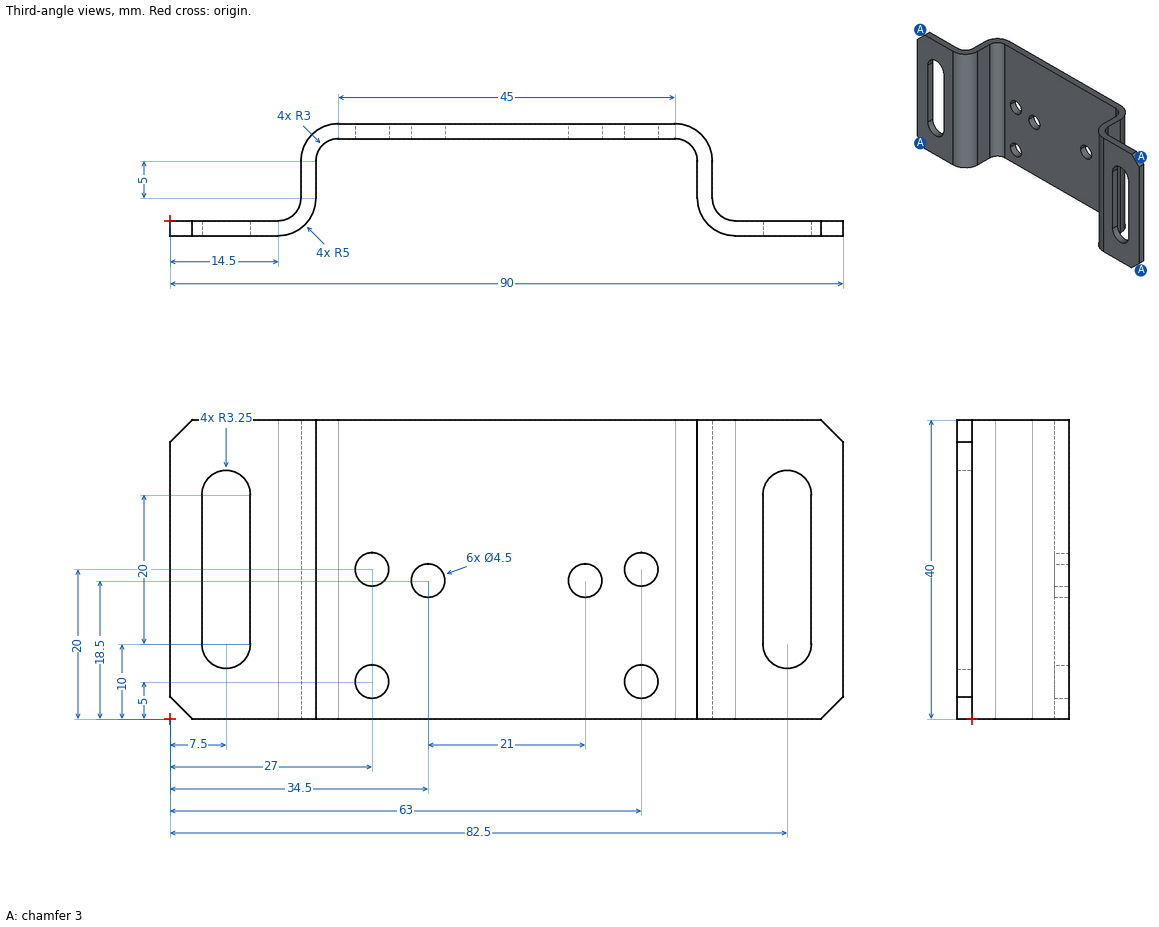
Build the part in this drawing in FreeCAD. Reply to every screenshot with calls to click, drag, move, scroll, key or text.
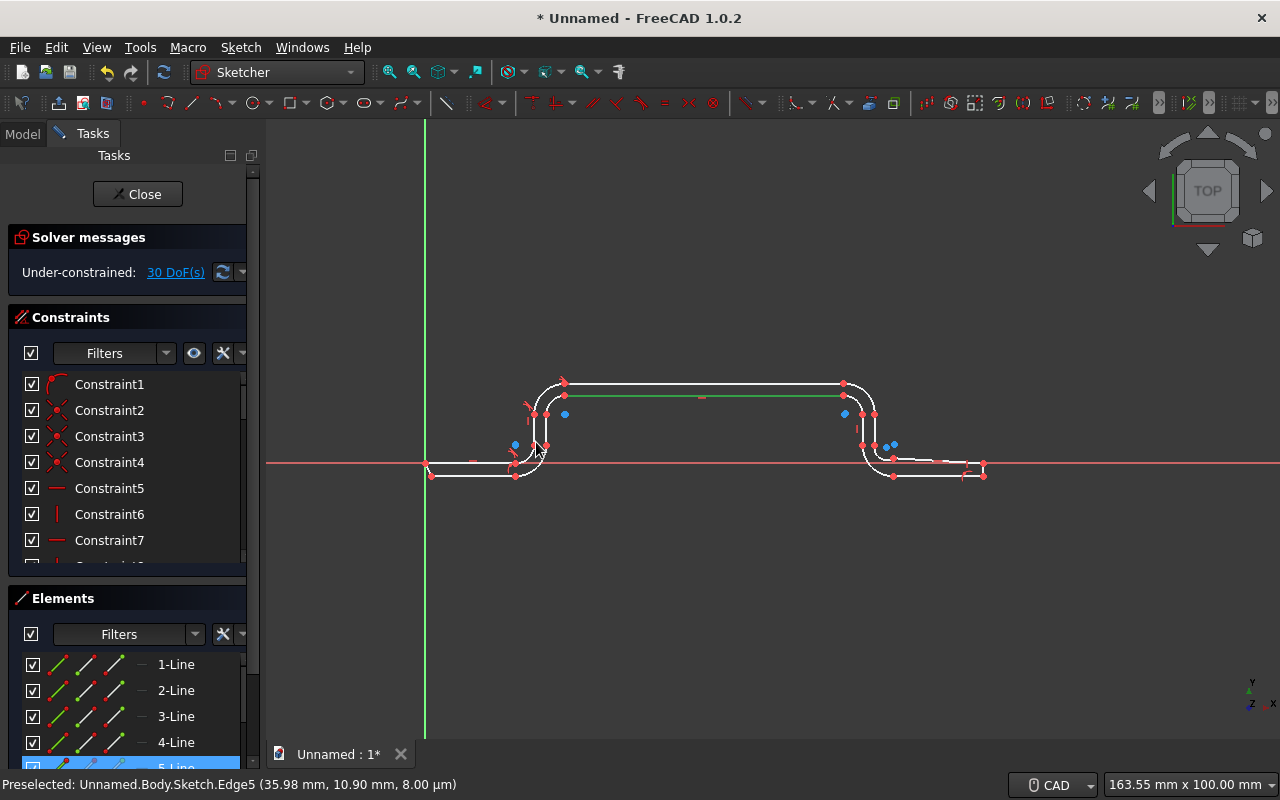
scroll(861, 406, up, 3)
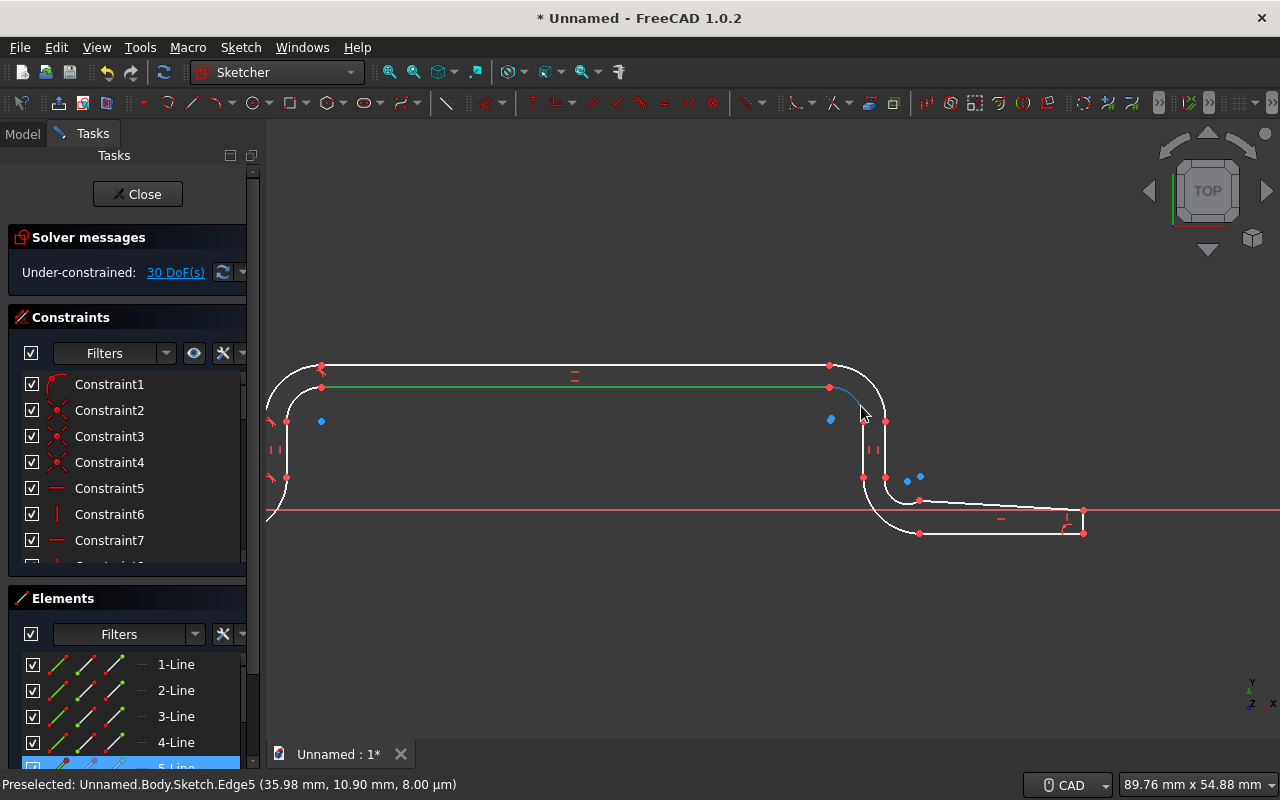
click(860, 406)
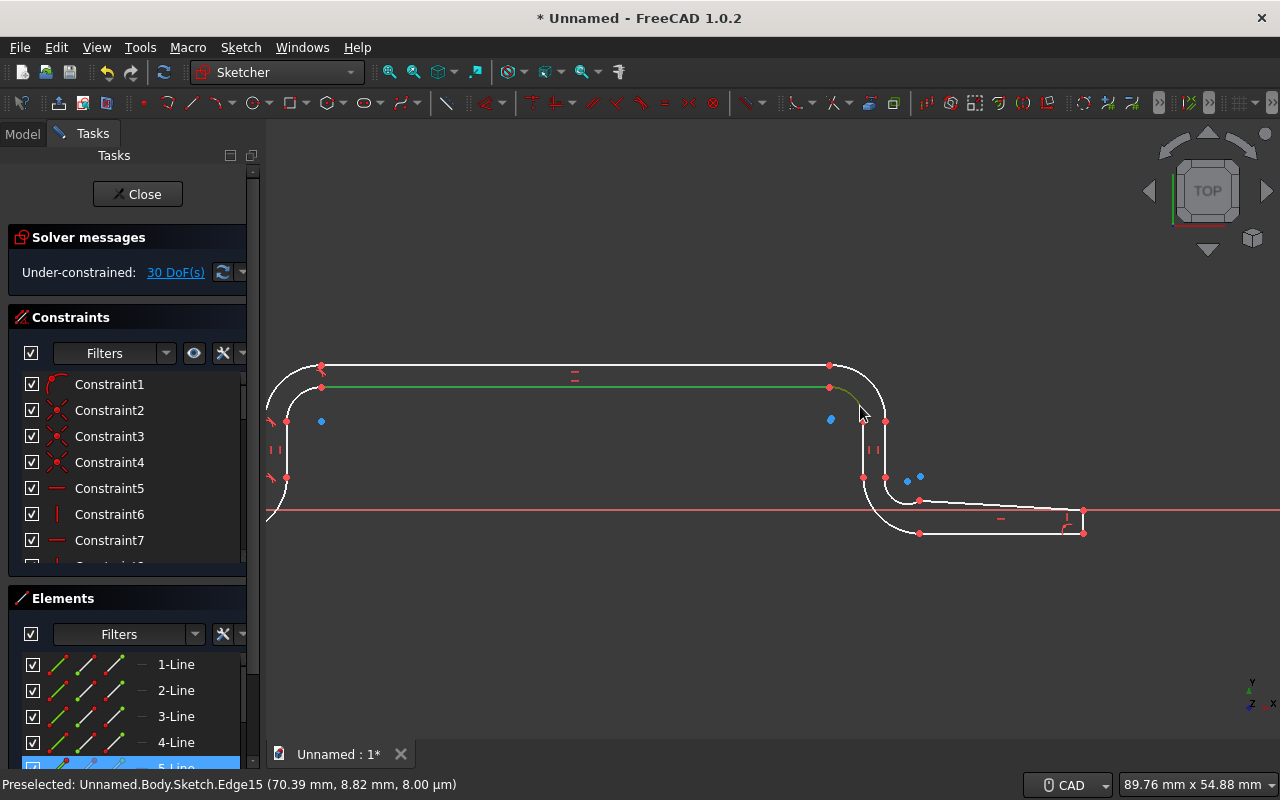
click(642, 104)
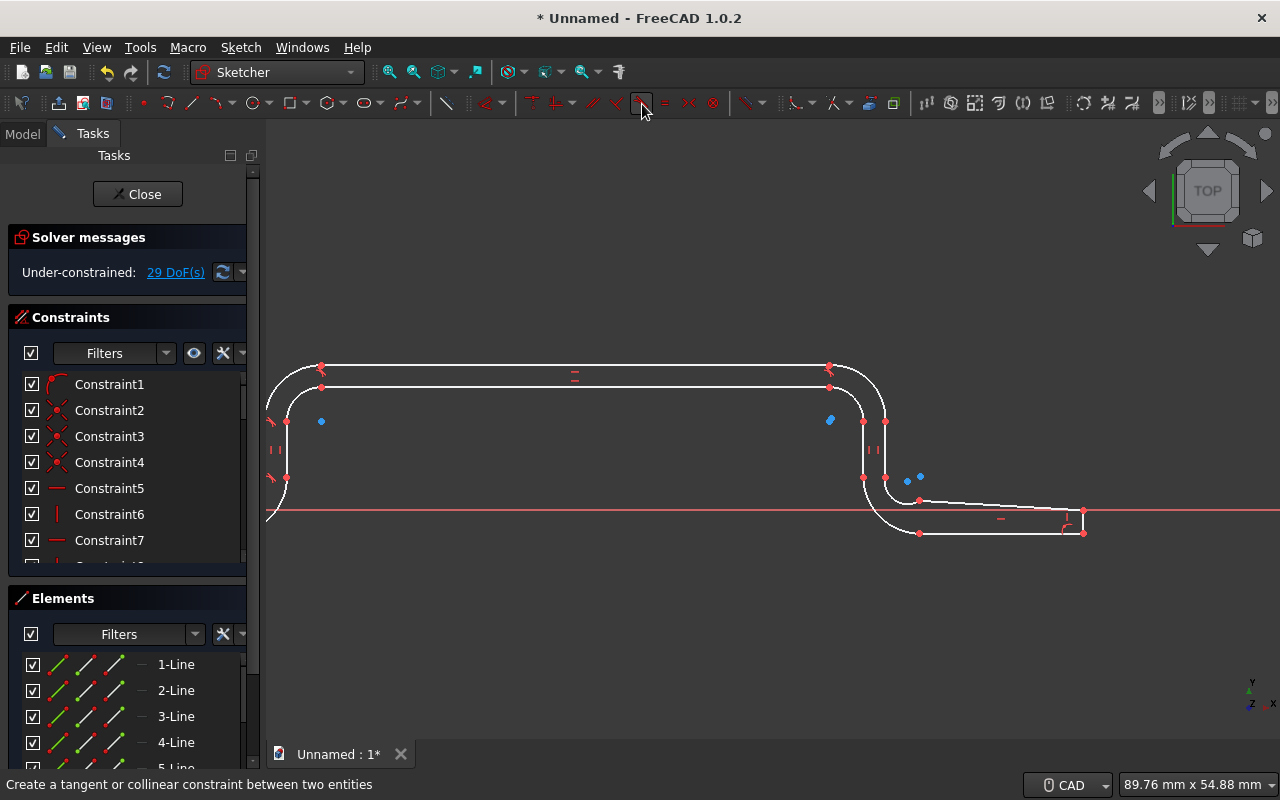
click(863, 438)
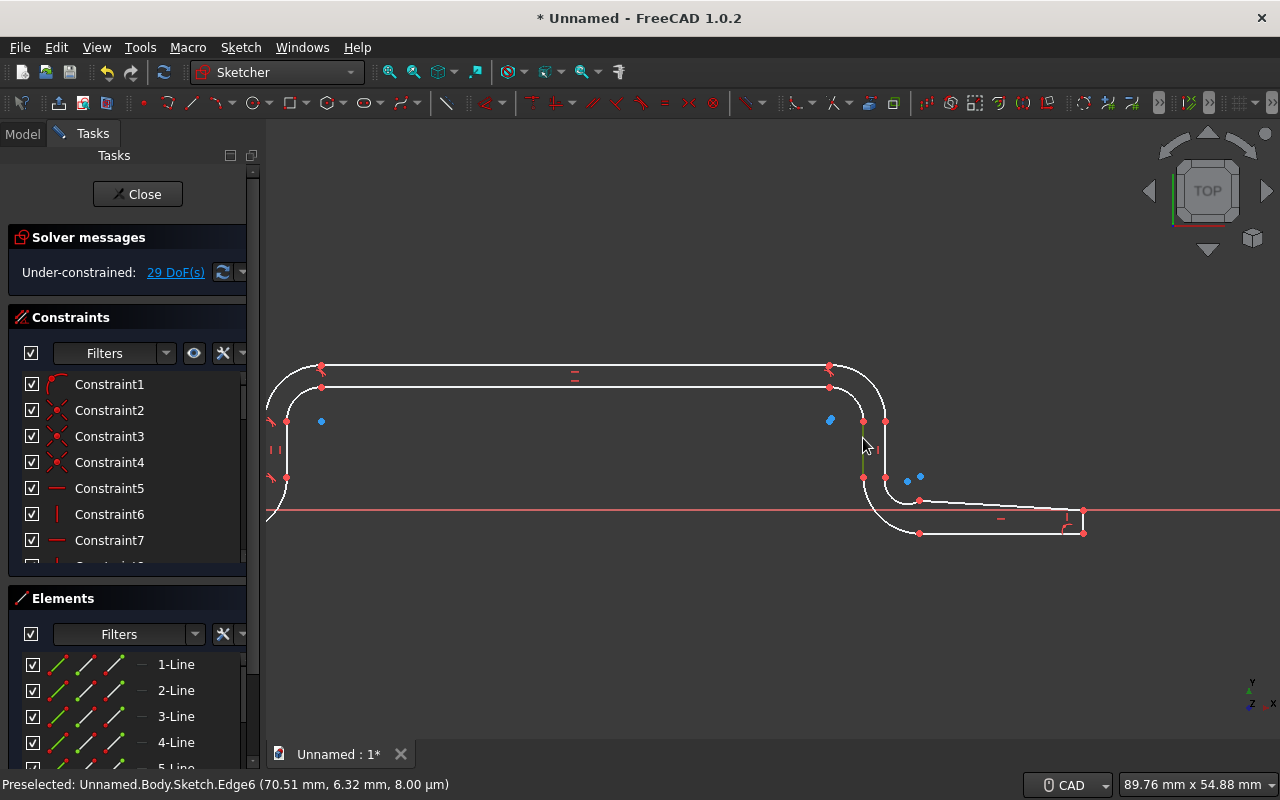
click(860, 406)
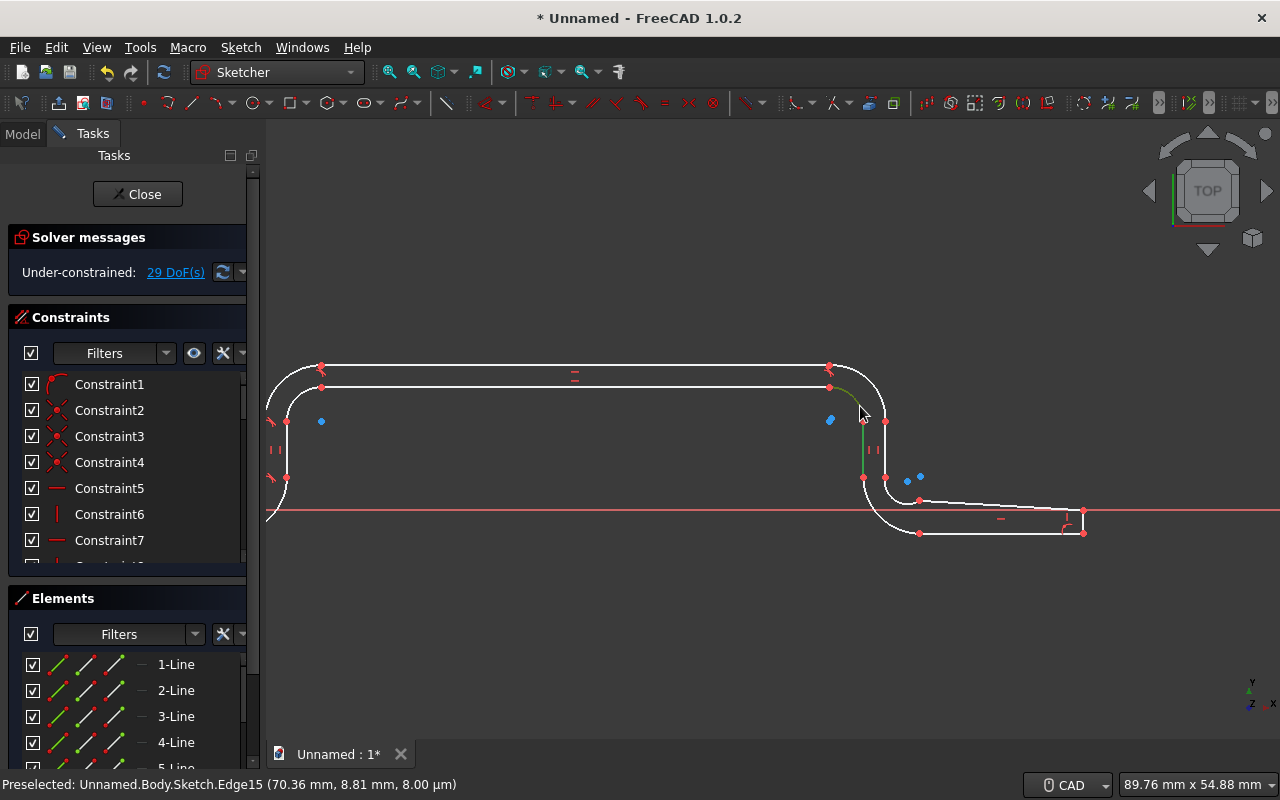
key(t)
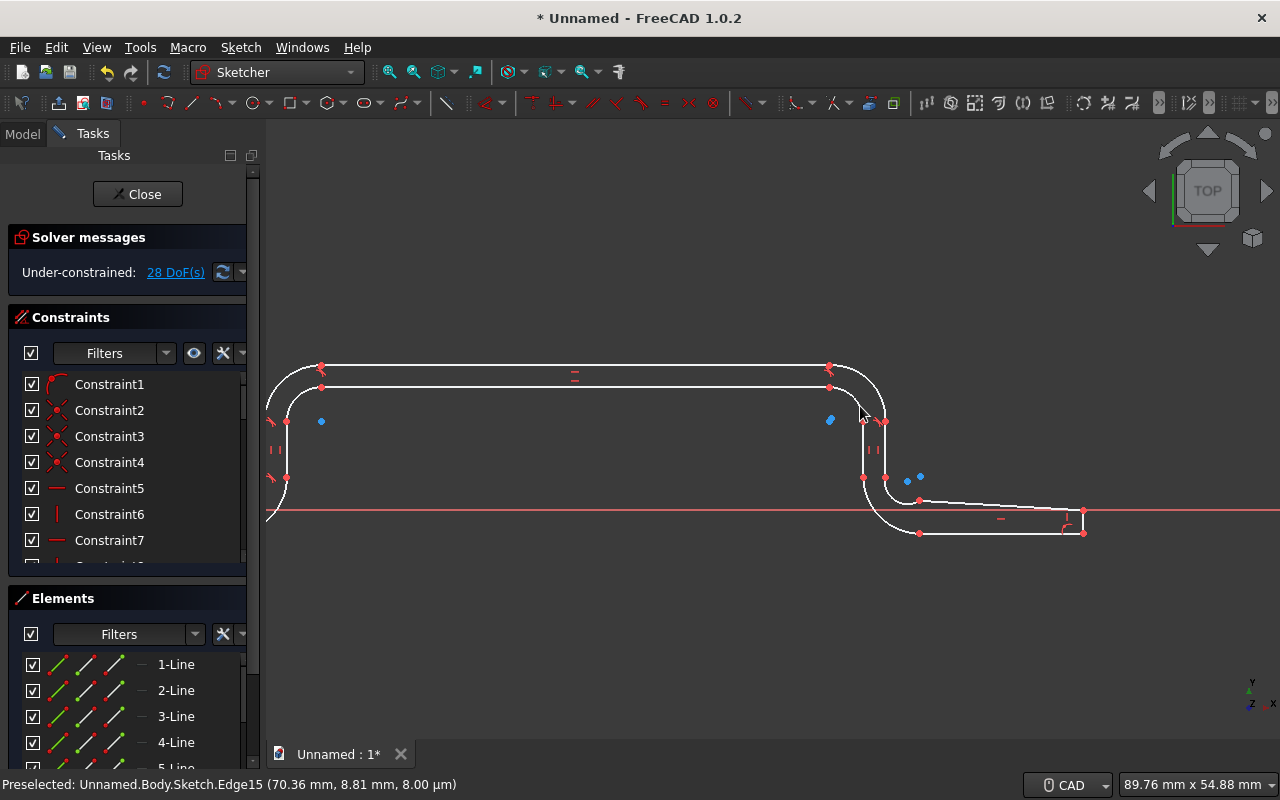
click(863, 438)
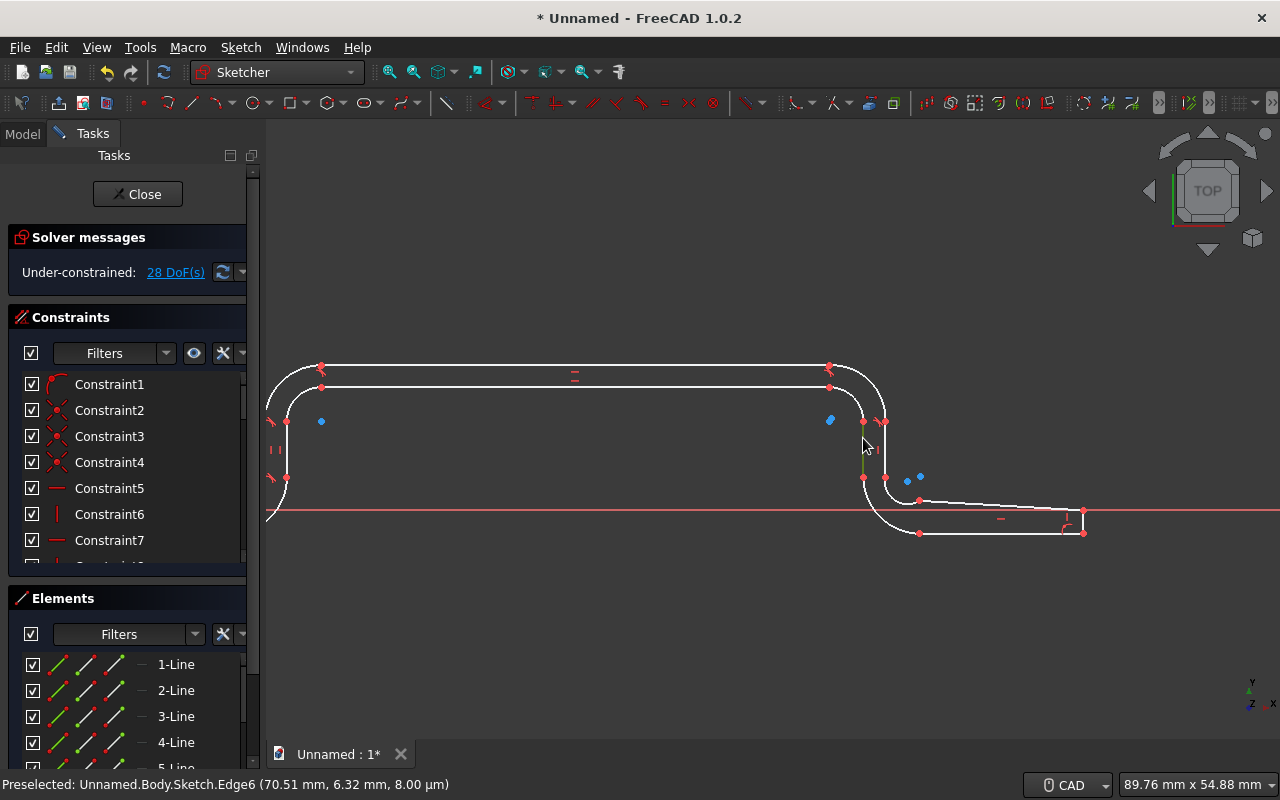
click(894, 527)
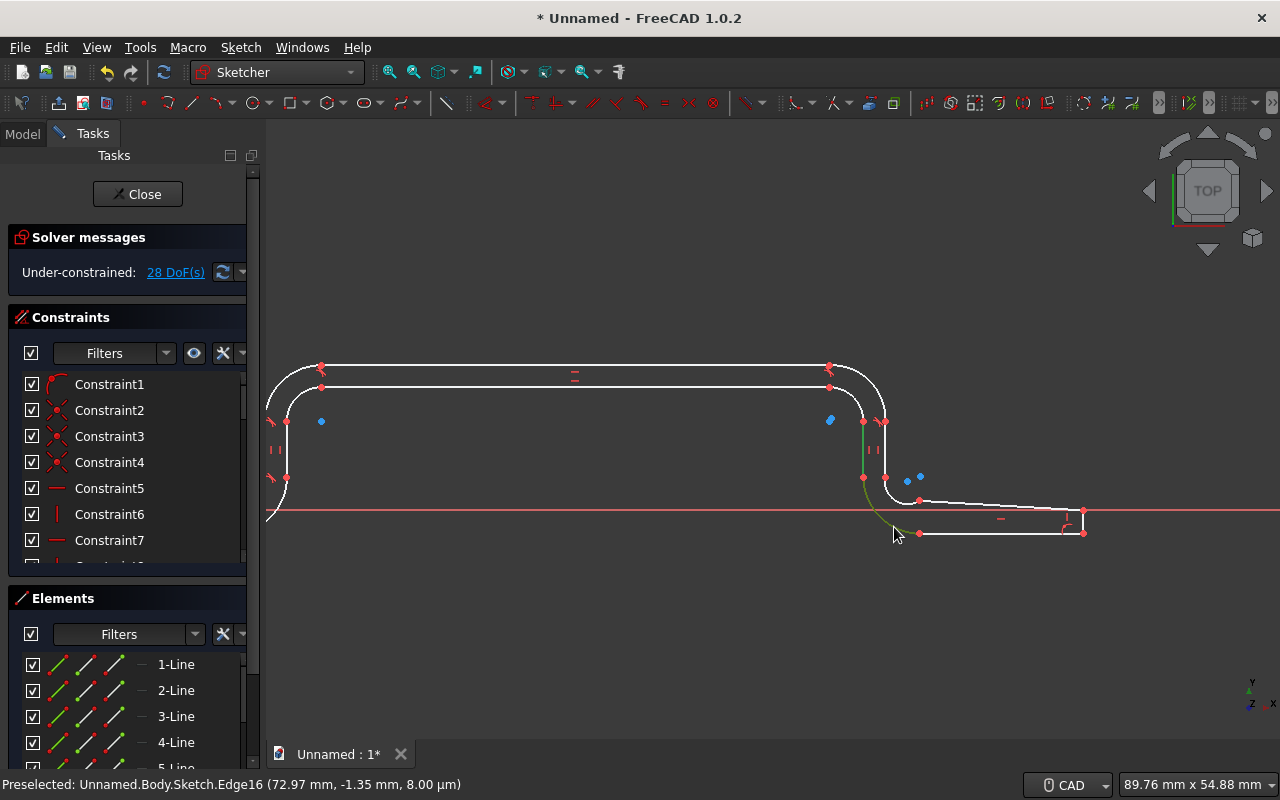
key(t)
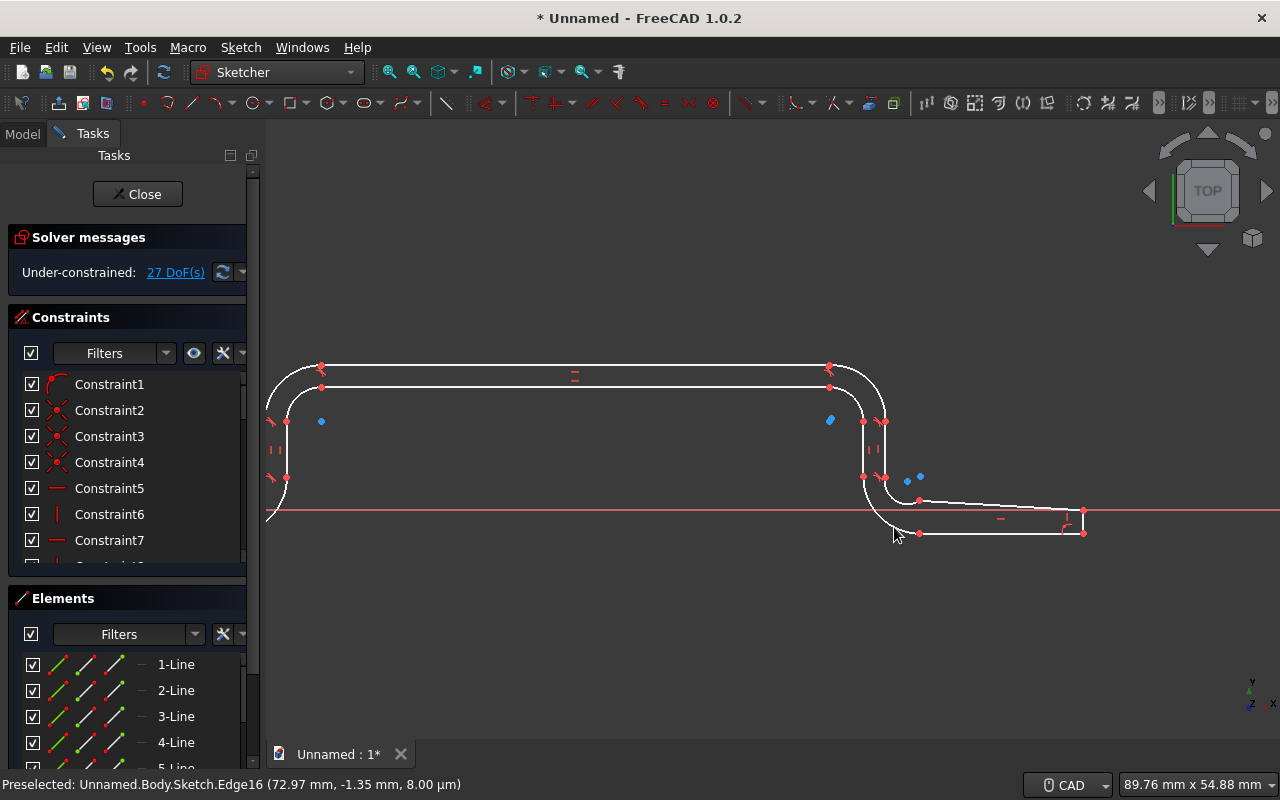
click(969, 534)